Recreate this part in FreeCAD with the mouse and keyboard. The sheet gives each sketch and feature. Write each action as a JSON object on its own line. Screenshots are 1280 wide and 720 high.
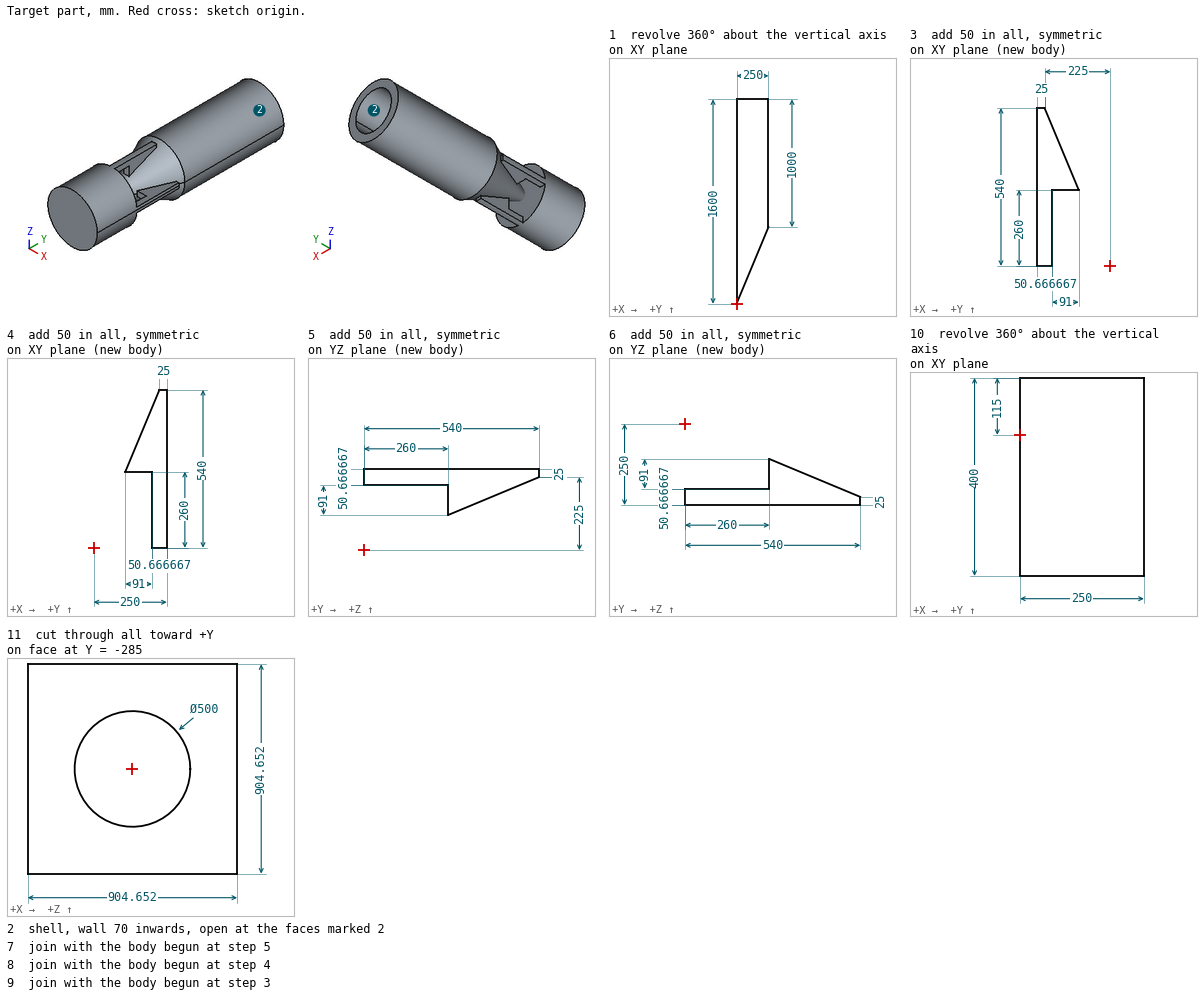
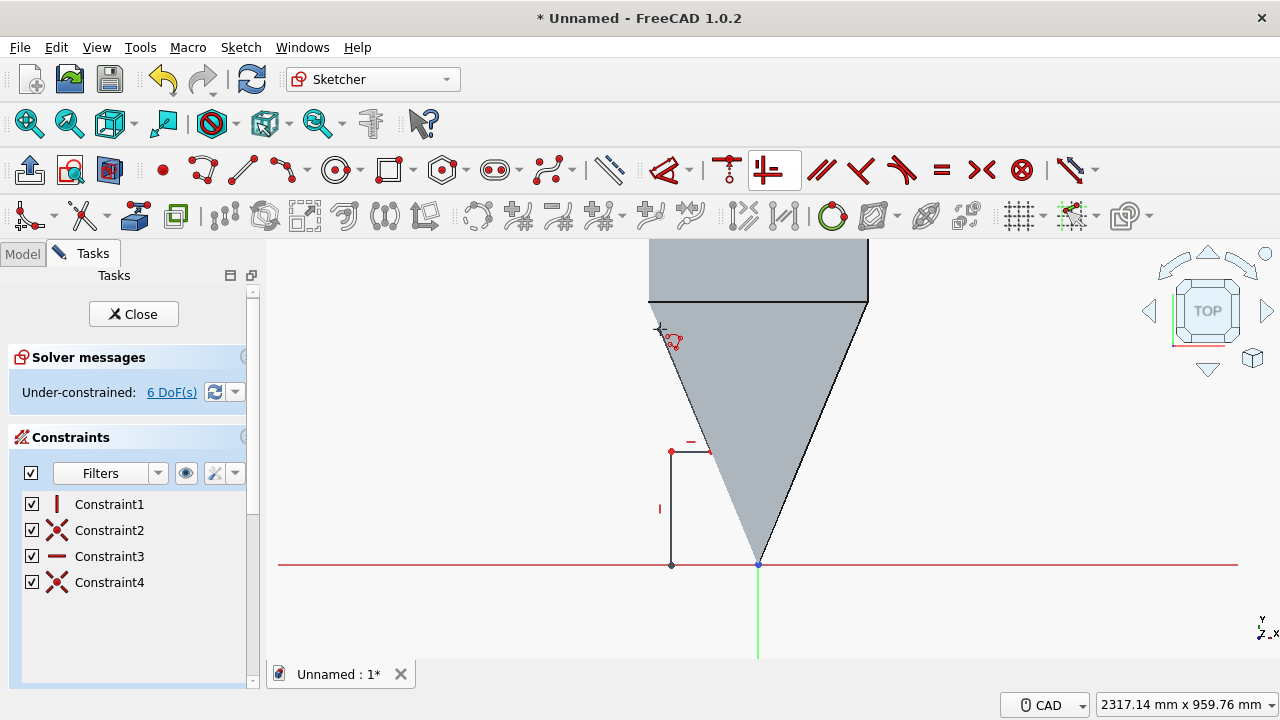
{"action": "scroll", "coordinate": [649, 329], "scroll_direction": "up", "scroll_amount": 2}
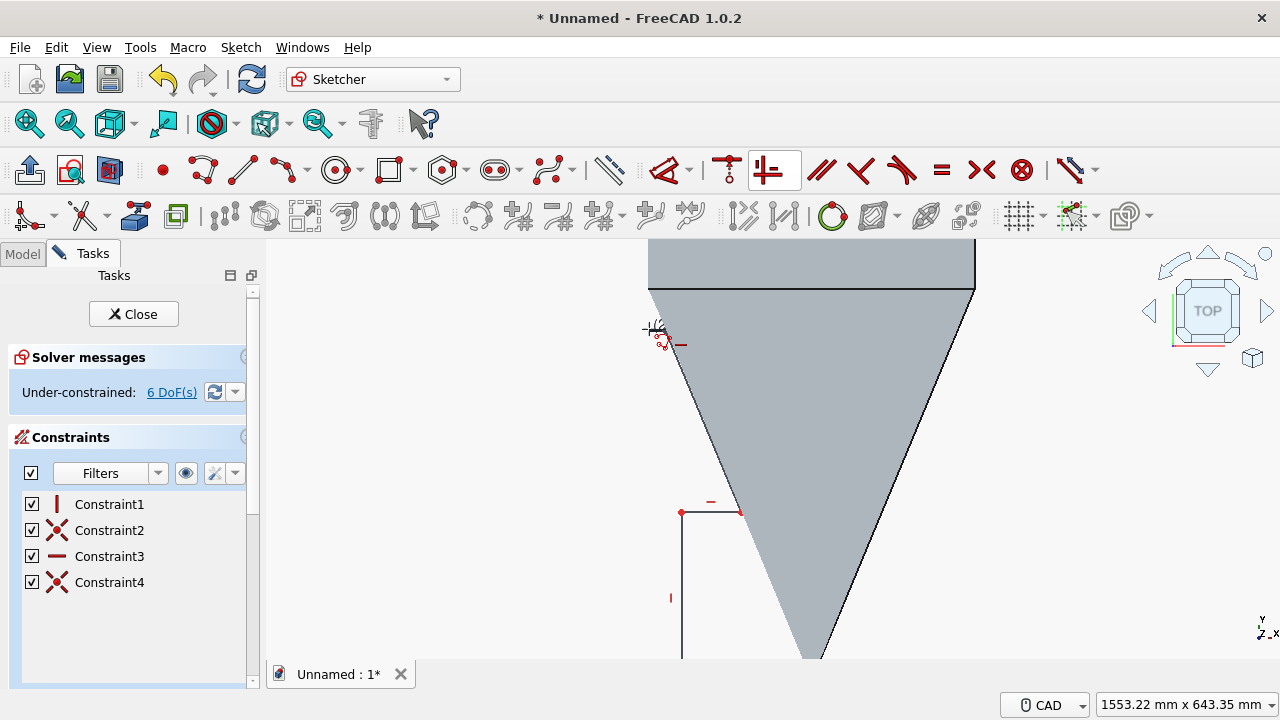
{"action": "left_click", "coordinate": [648, 329]}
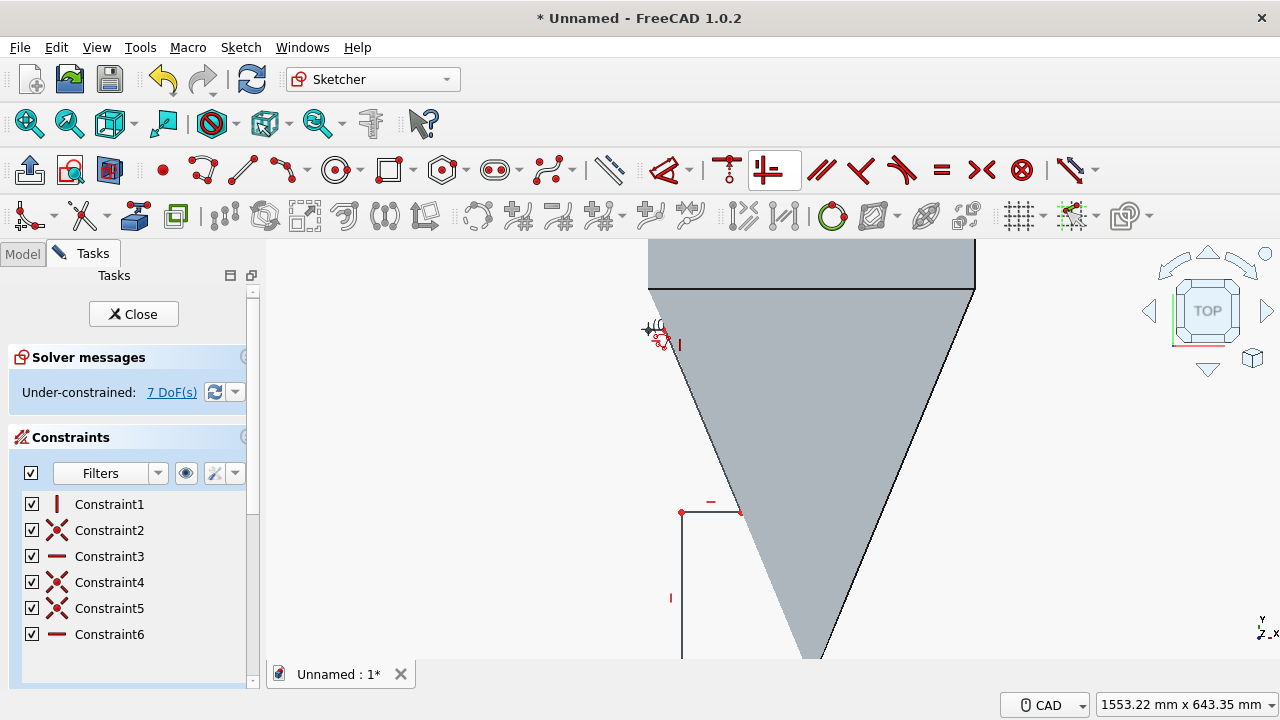
{"action": "scroll", "coordinate": [653, 336], "scroll_direction": "down", "scroll_amount": 2}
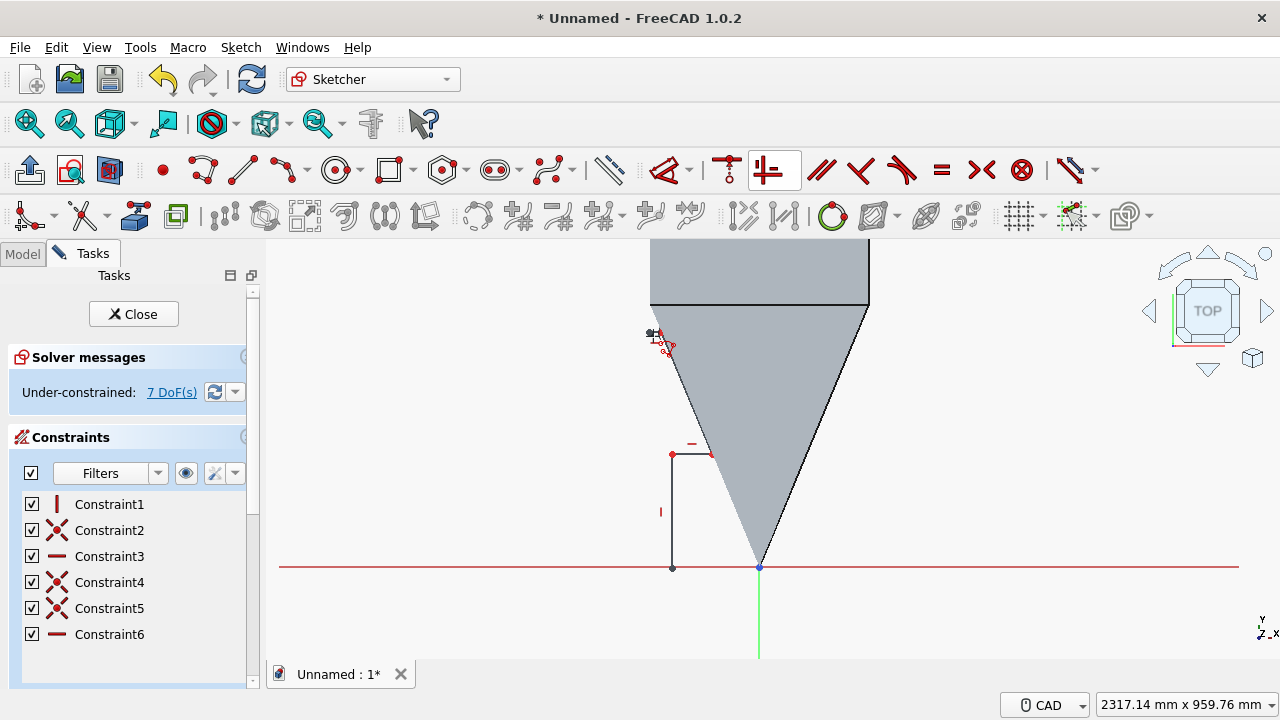
{"action": "left_click", "coordinate": [650, 558]}
{"action": "left_click", "coordinate": [672, 568]}
{"action": "key", "text": "Escape"}
{"action": "key", "text": "Escape"}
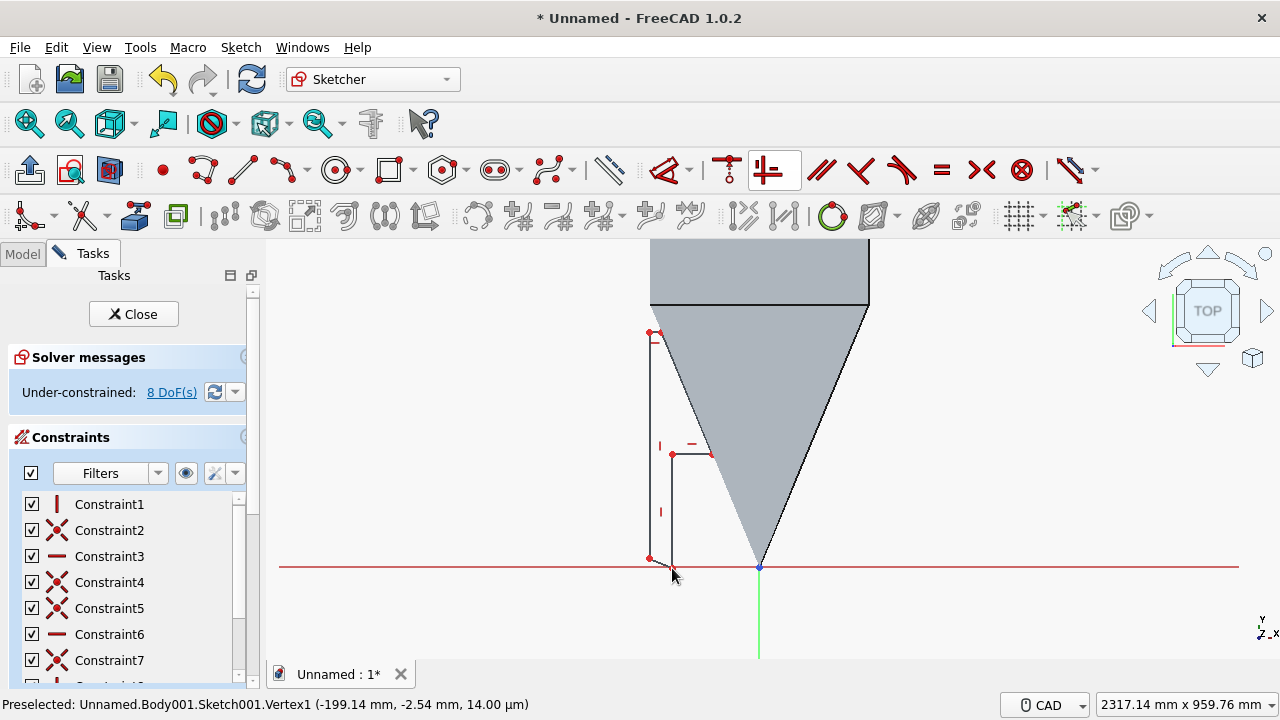
{"action": "scroll", "coordinate": [663, 565], "scroll_direction": "up", "scroll_amount": 3}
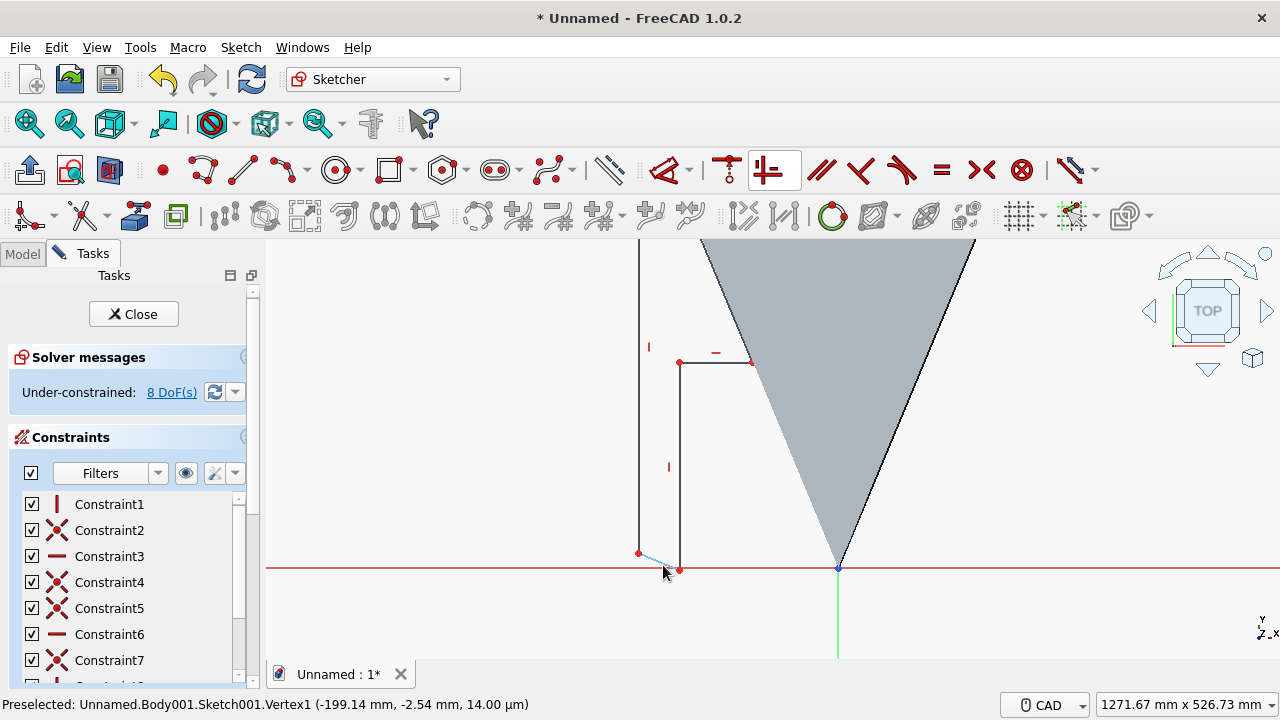
{"action": "left_click", "coordinate": [663, 564]}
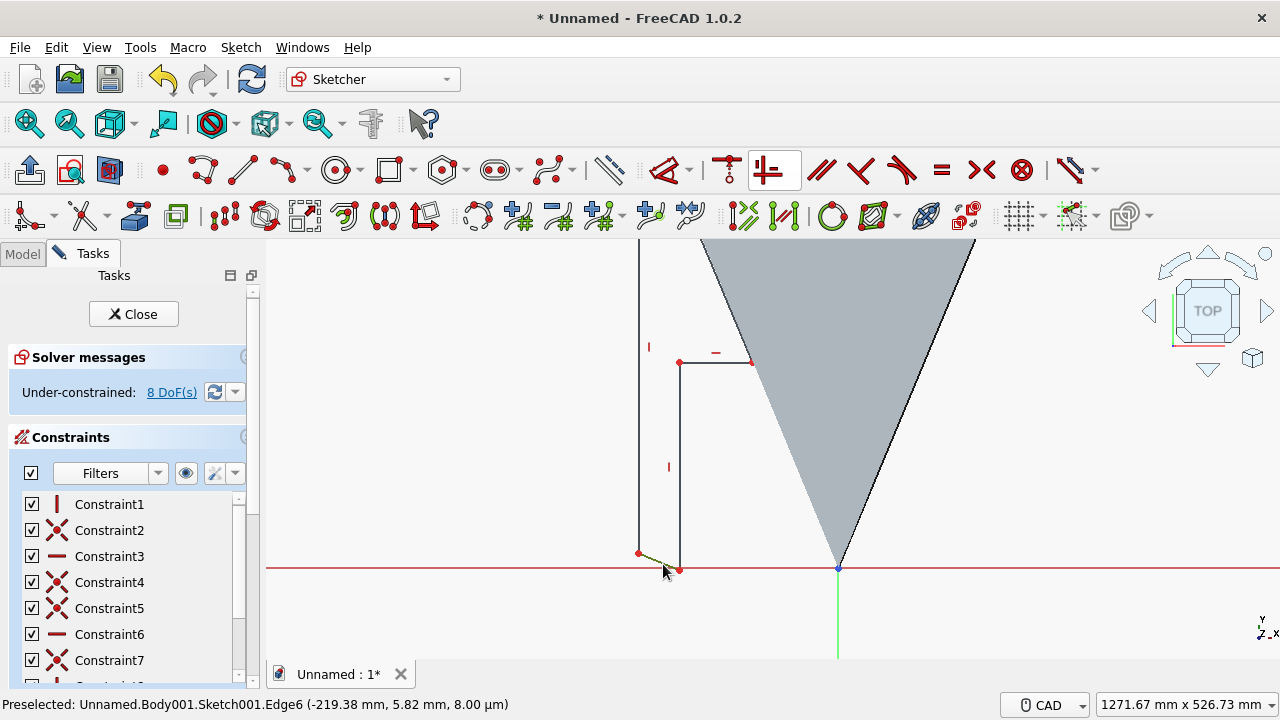
{"action": "left_click", "coordinate": [796, 170]}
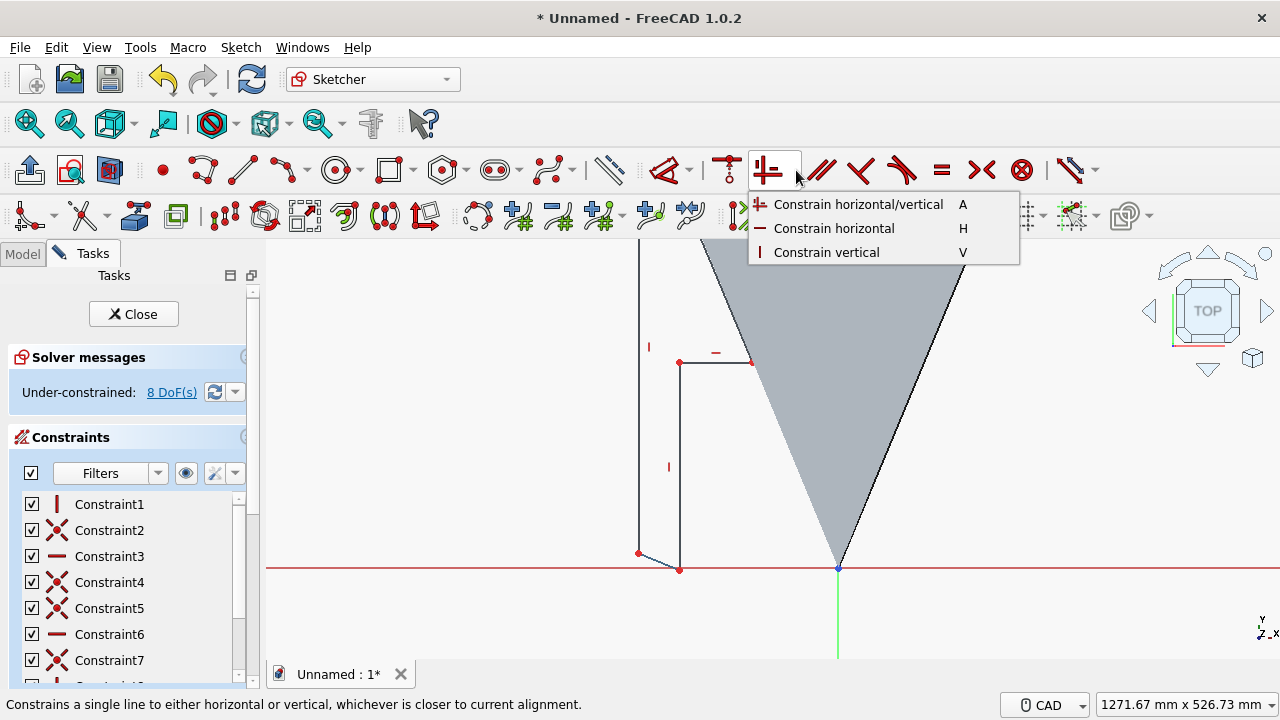
{"action": "left_click", "coordinate": [884, 228]}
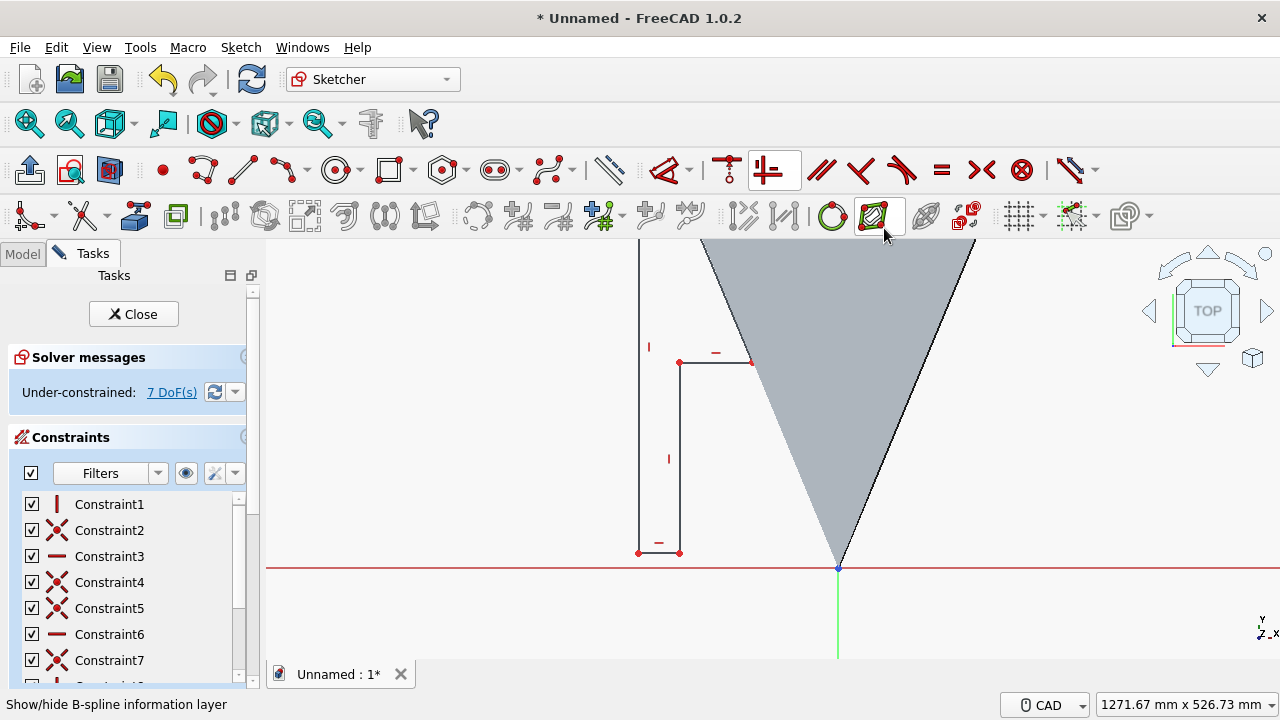
{"action": "left_click", "coordinate": [680, 553]}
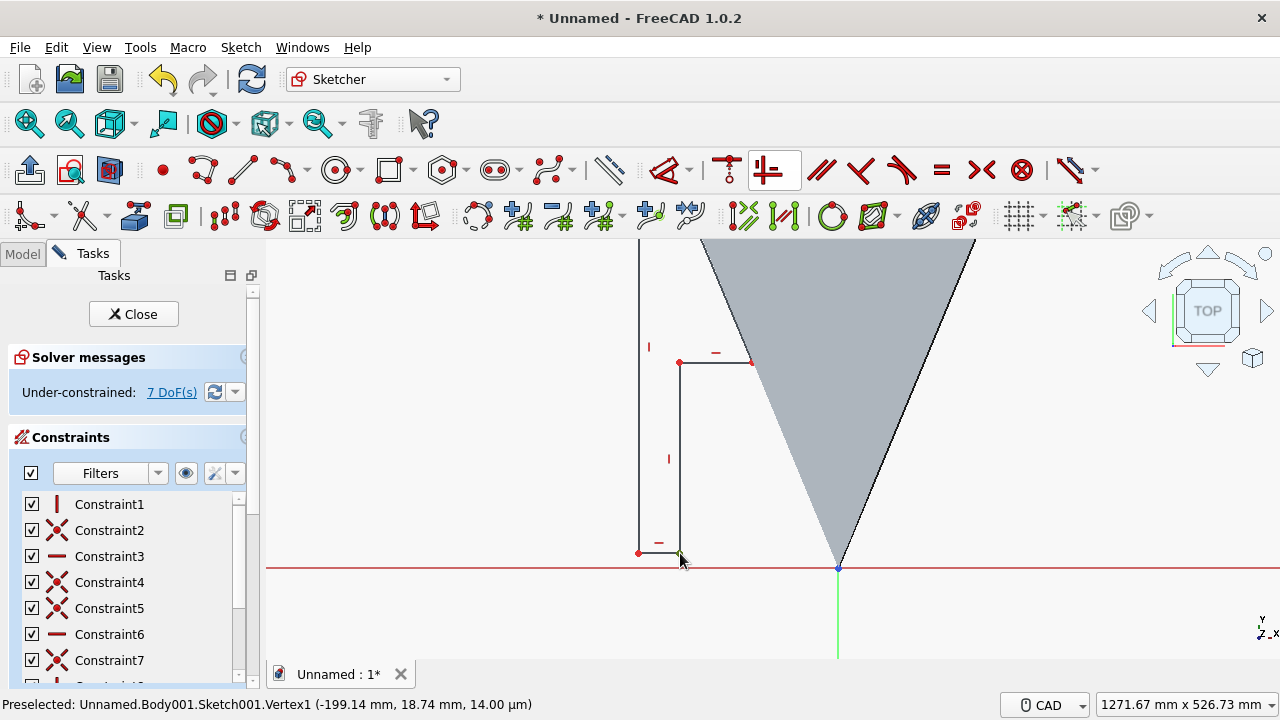
{"action": "left_click", "coordinate": [353, 568]}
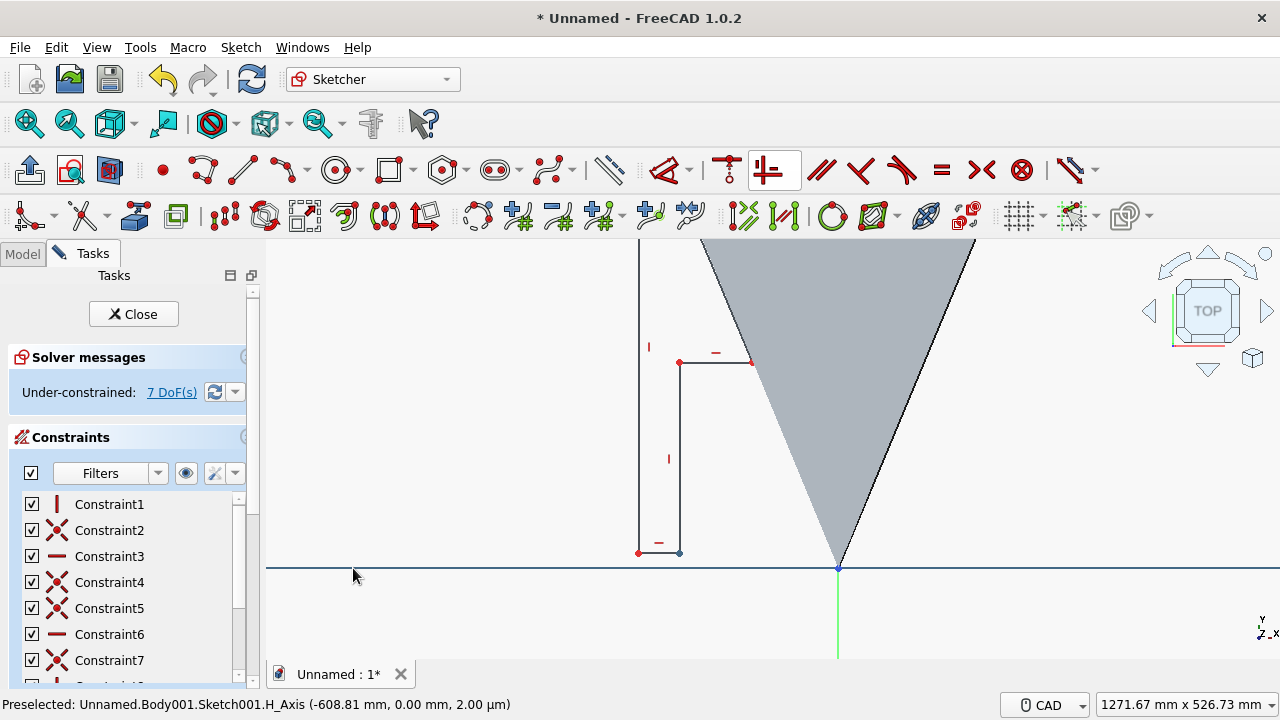
{"action": "left_click", "coordinate": [728, 170]}